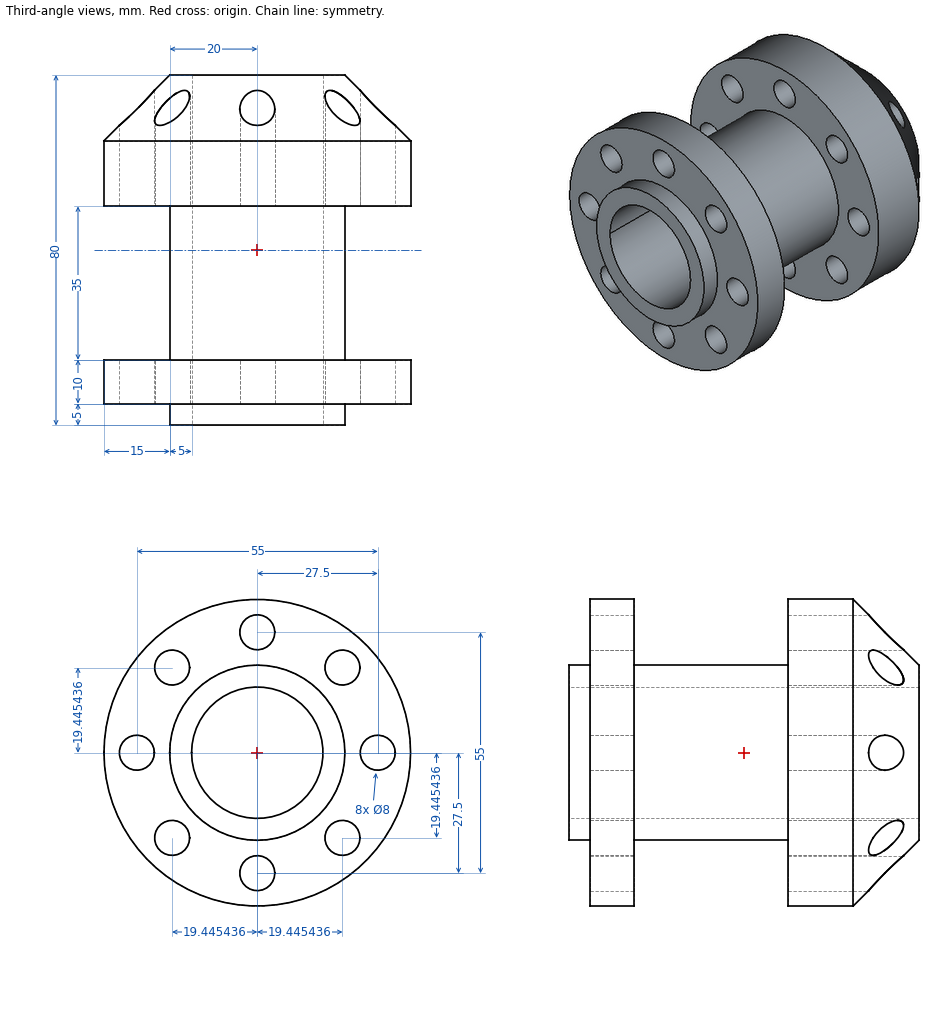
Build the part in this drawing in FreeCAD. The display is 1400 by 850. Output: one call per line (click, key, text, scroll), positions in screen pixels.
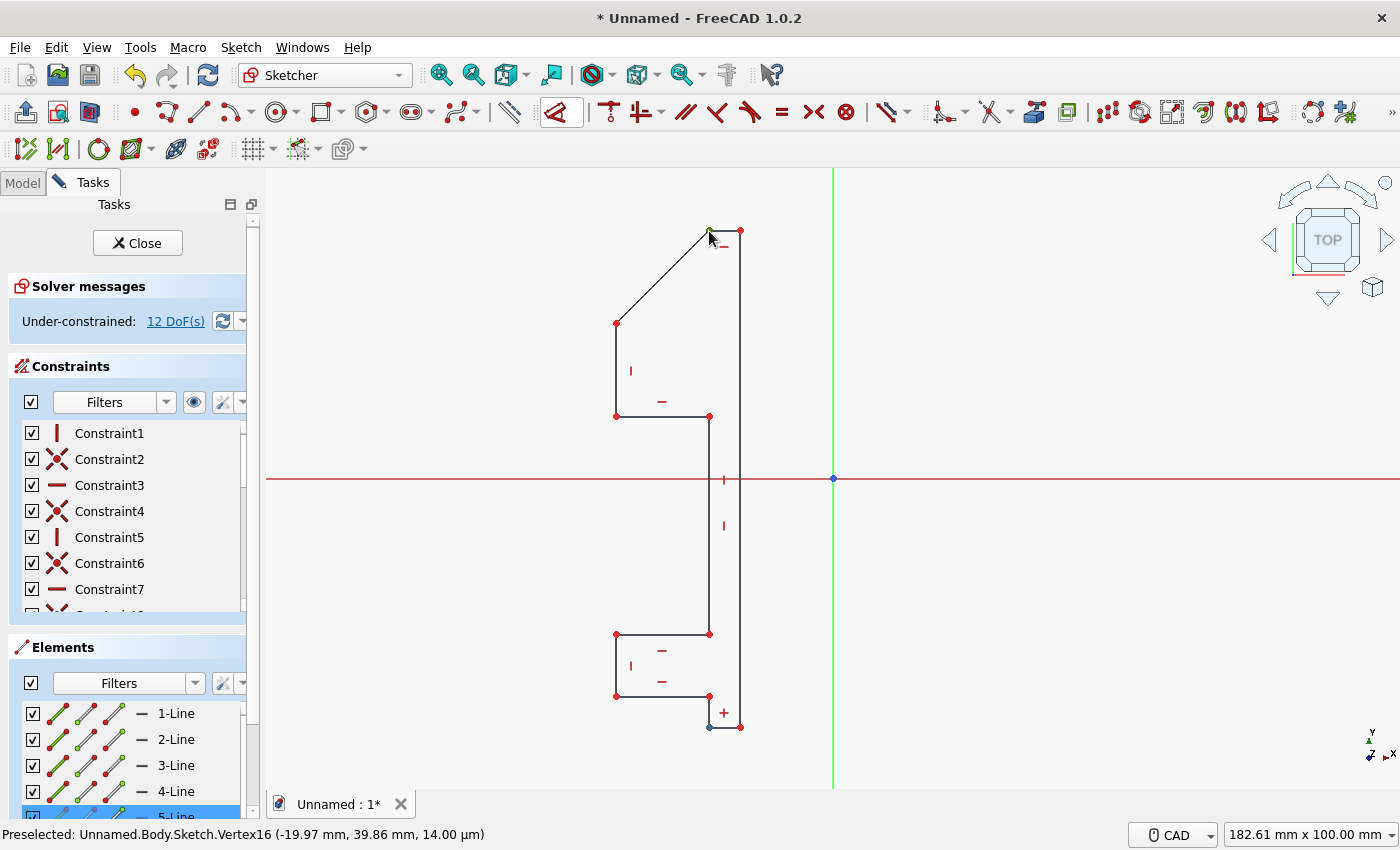
click(361, 478)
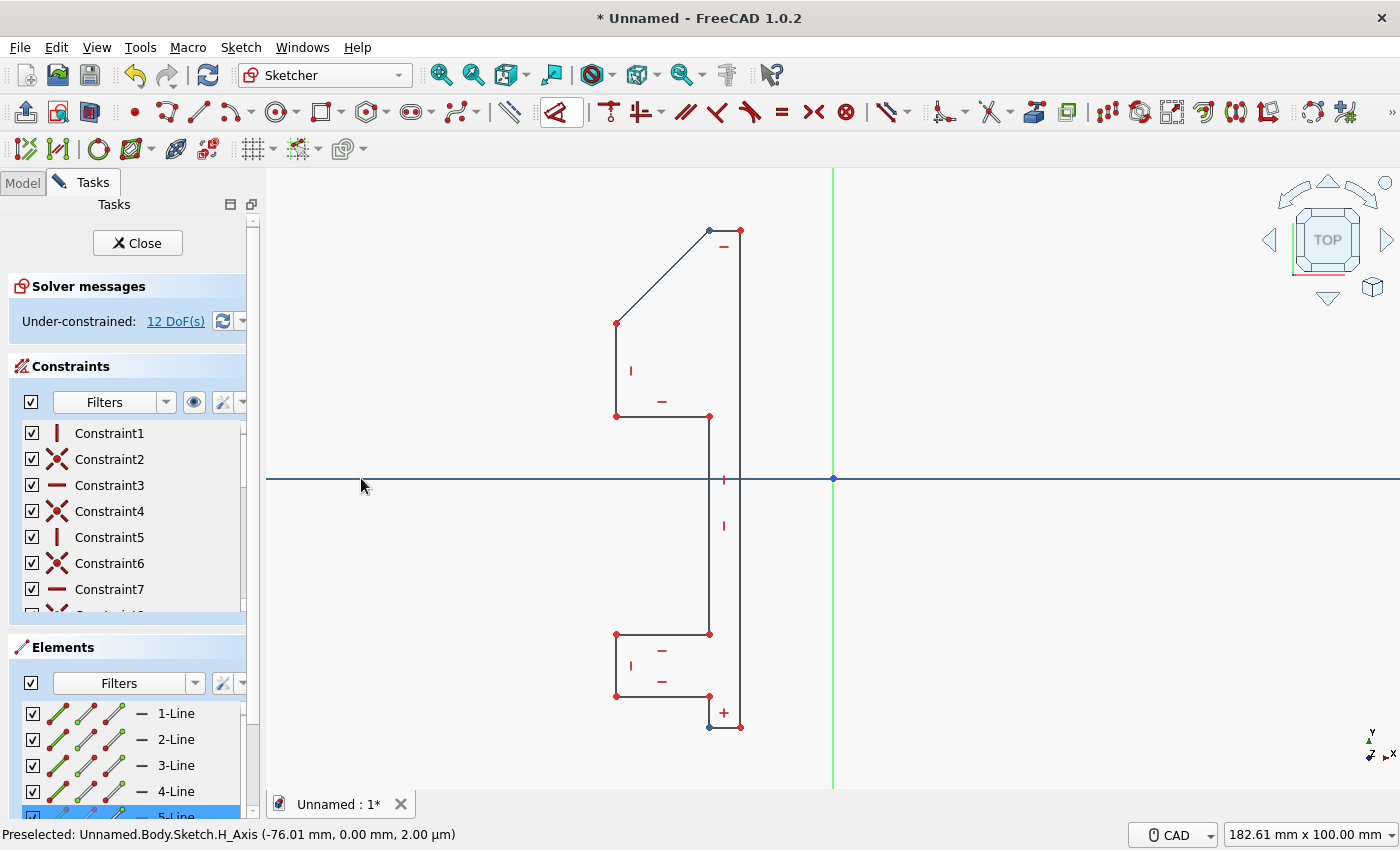
click(814, 112)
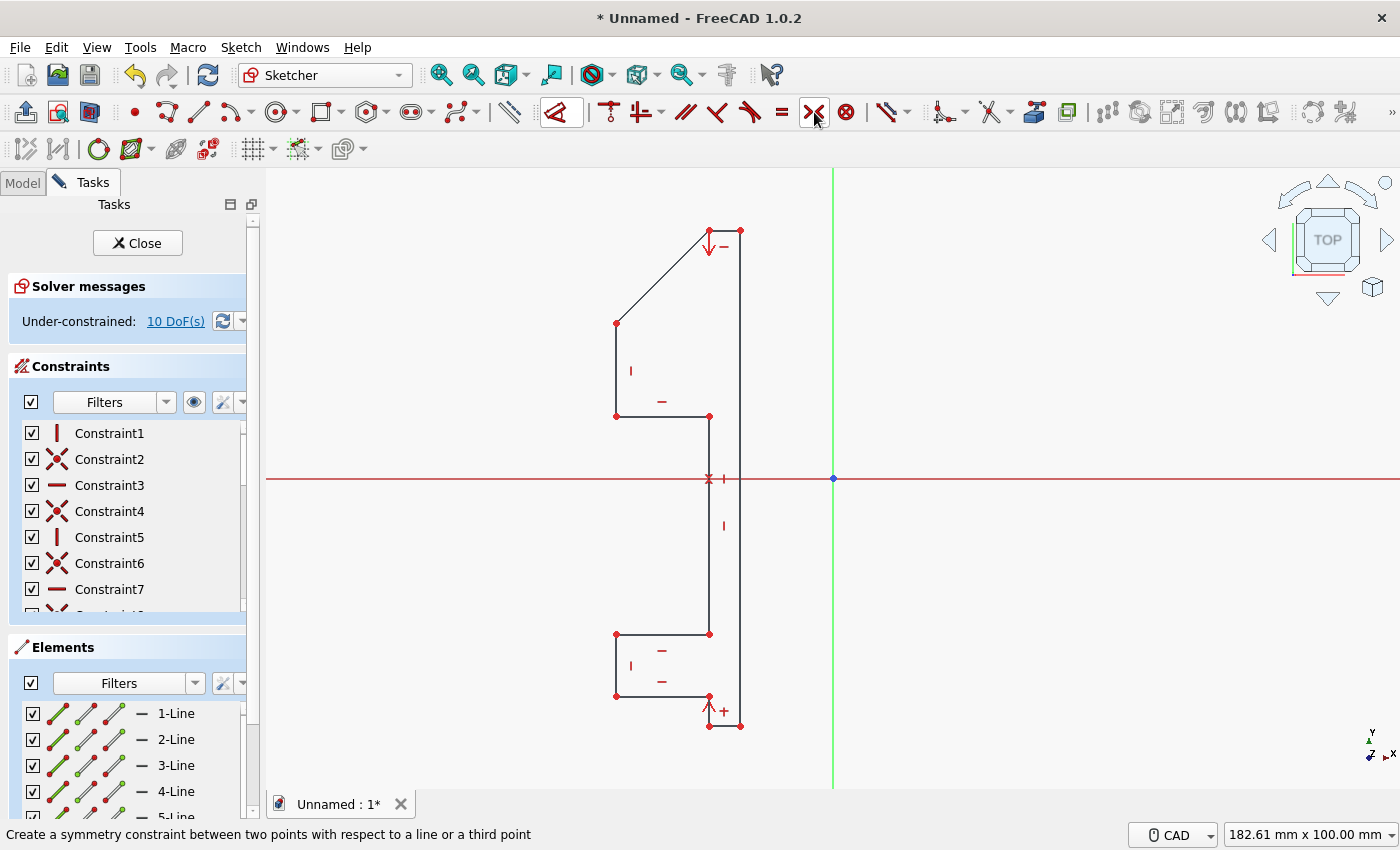
click(616, 635)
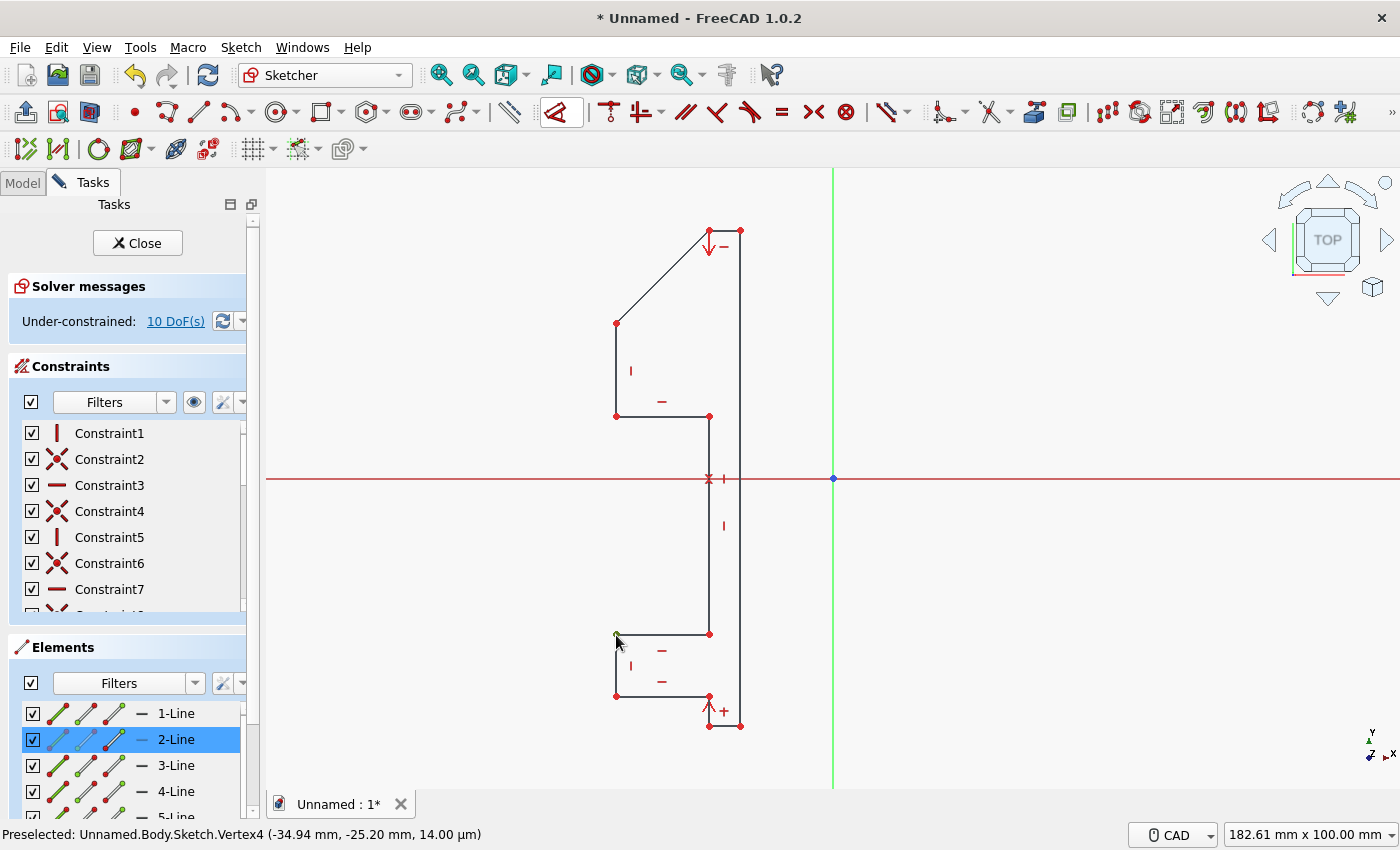
click(616, 324)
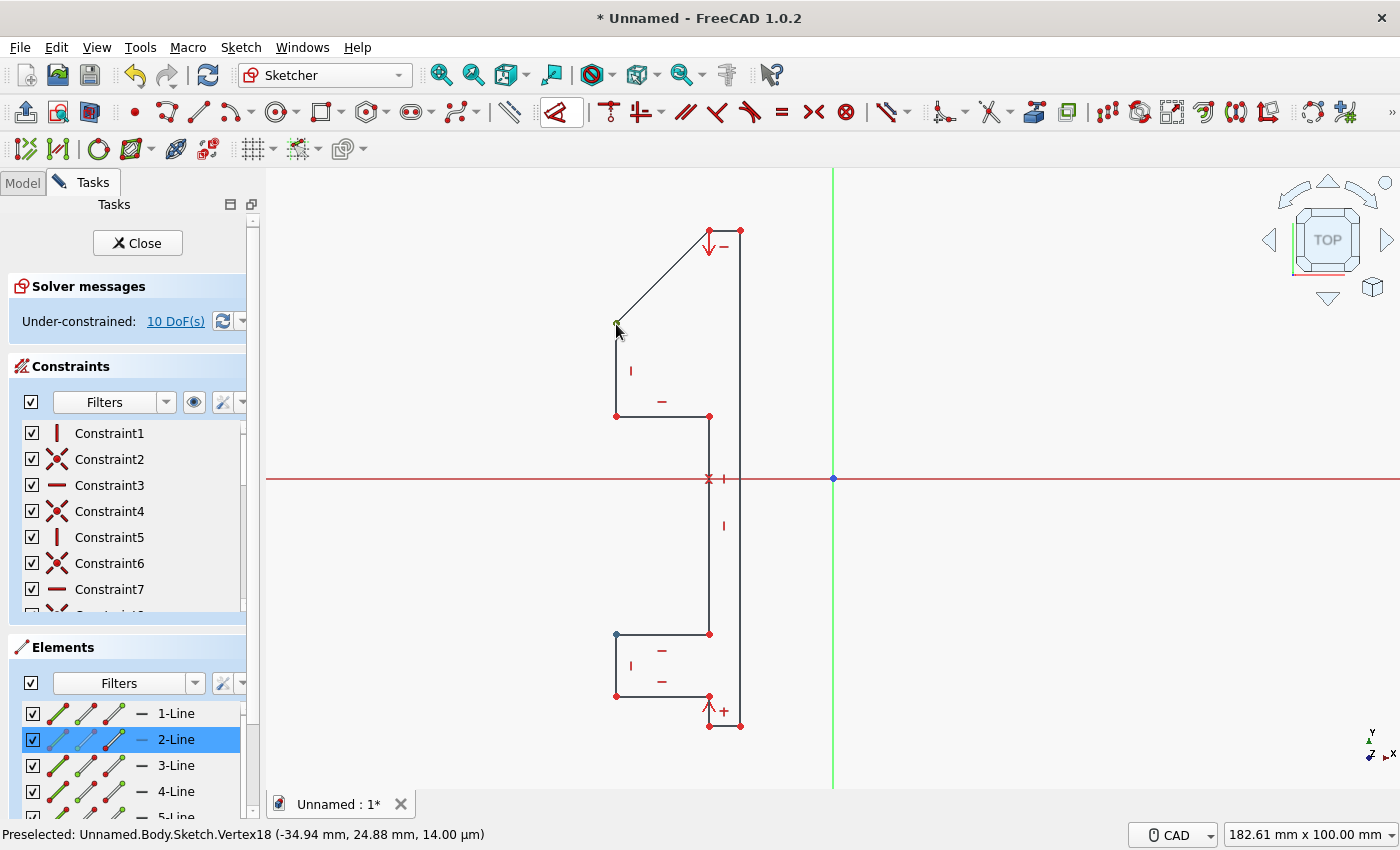
click(361, 478)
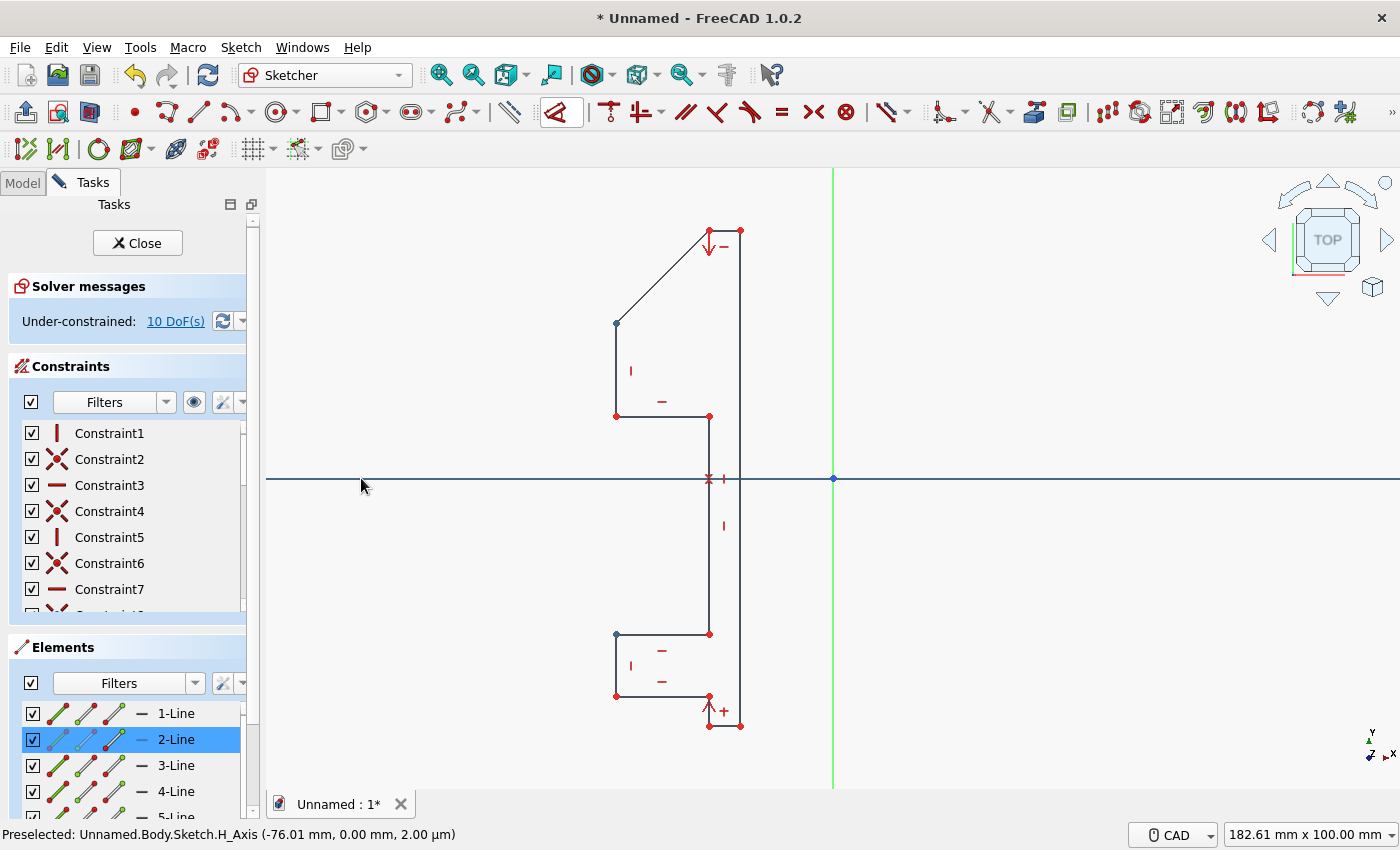
click(814, 112)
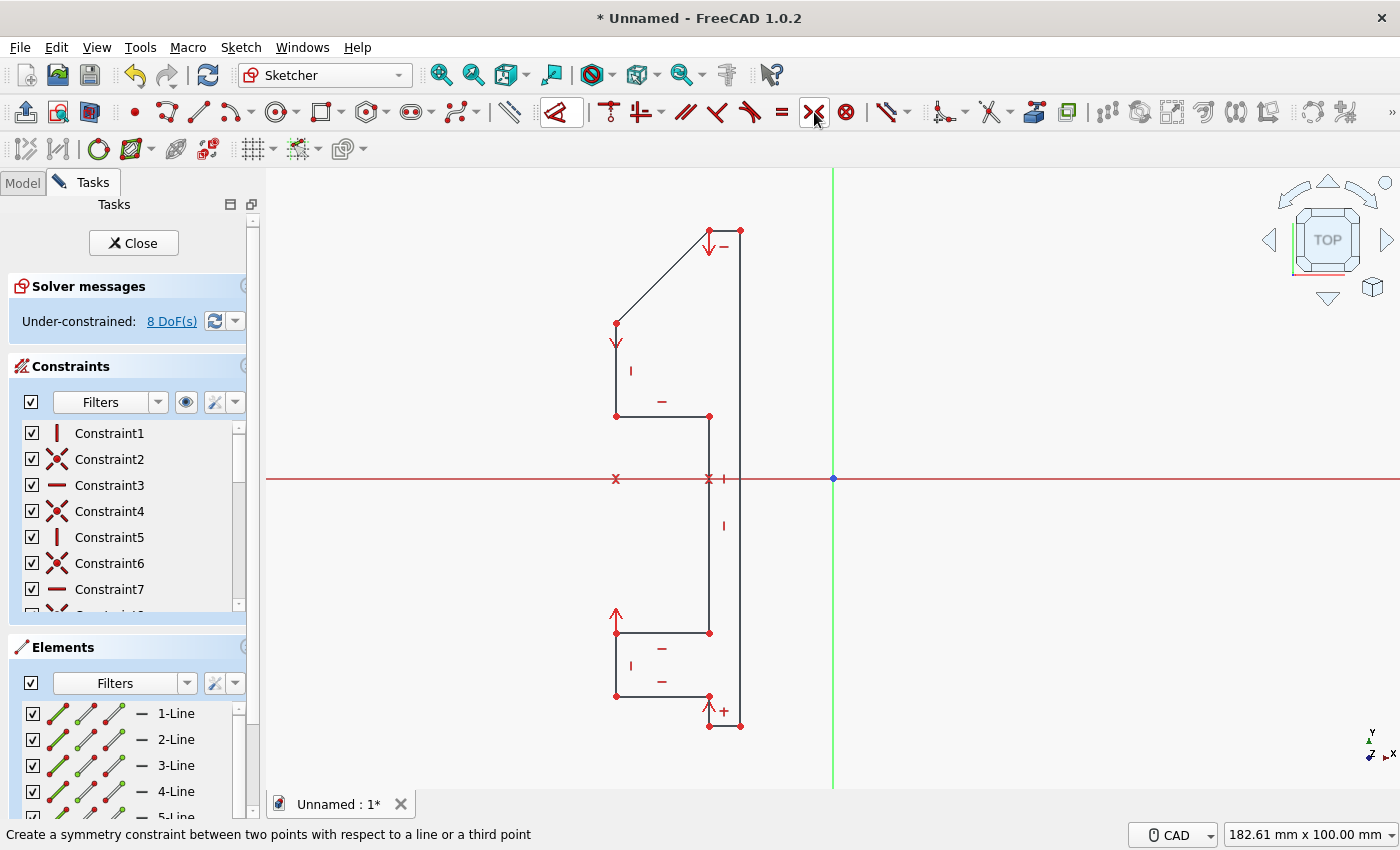
click(556, 112)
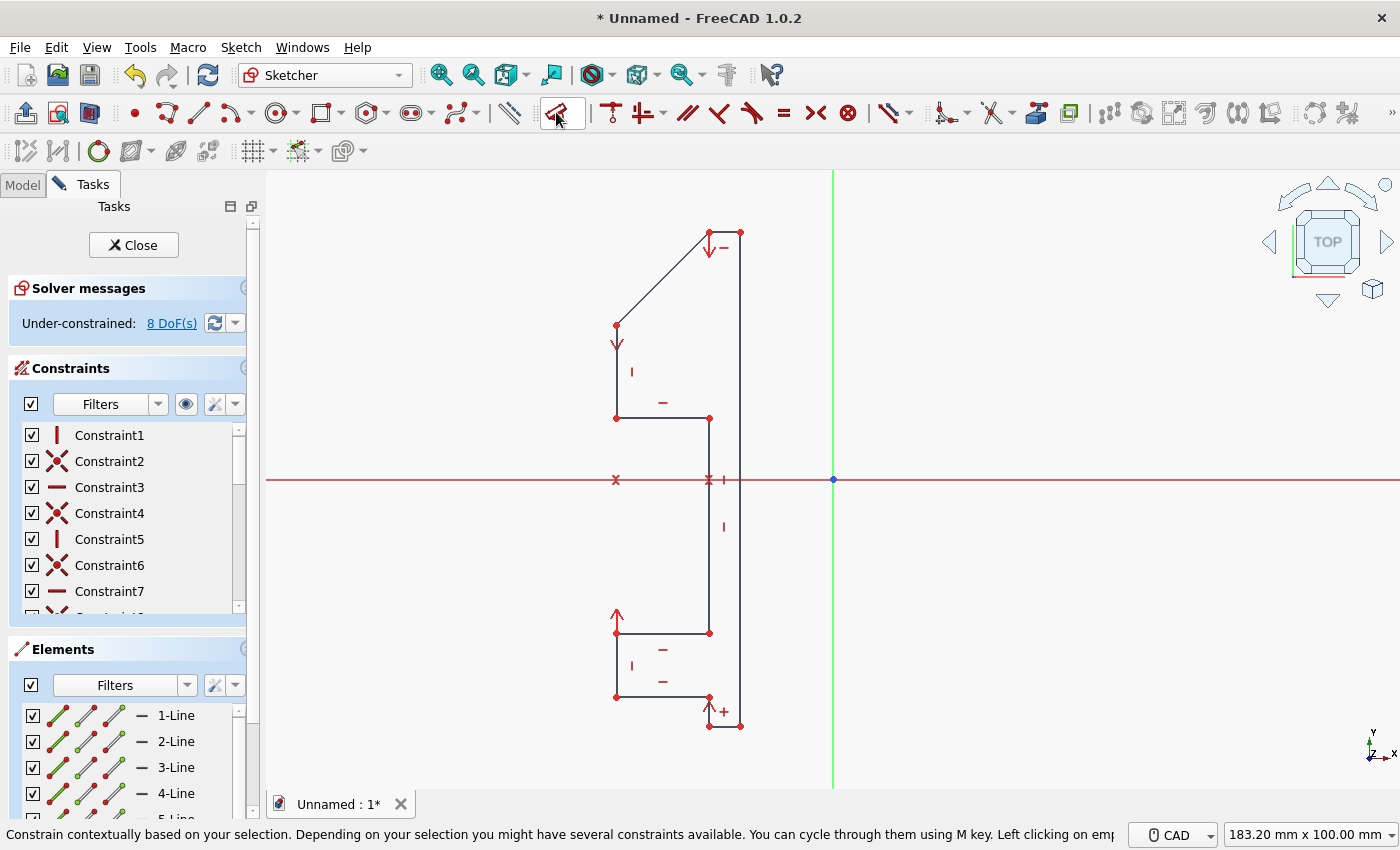
scroll(709, 709, up, 2)